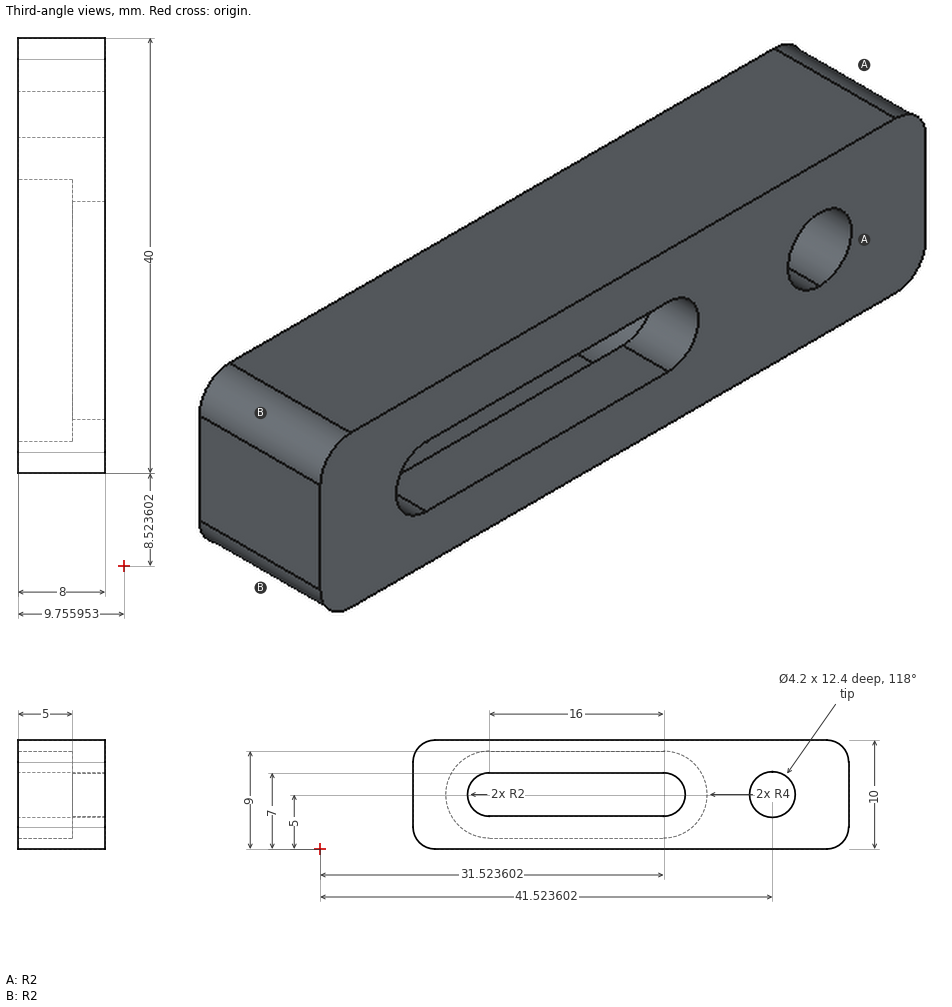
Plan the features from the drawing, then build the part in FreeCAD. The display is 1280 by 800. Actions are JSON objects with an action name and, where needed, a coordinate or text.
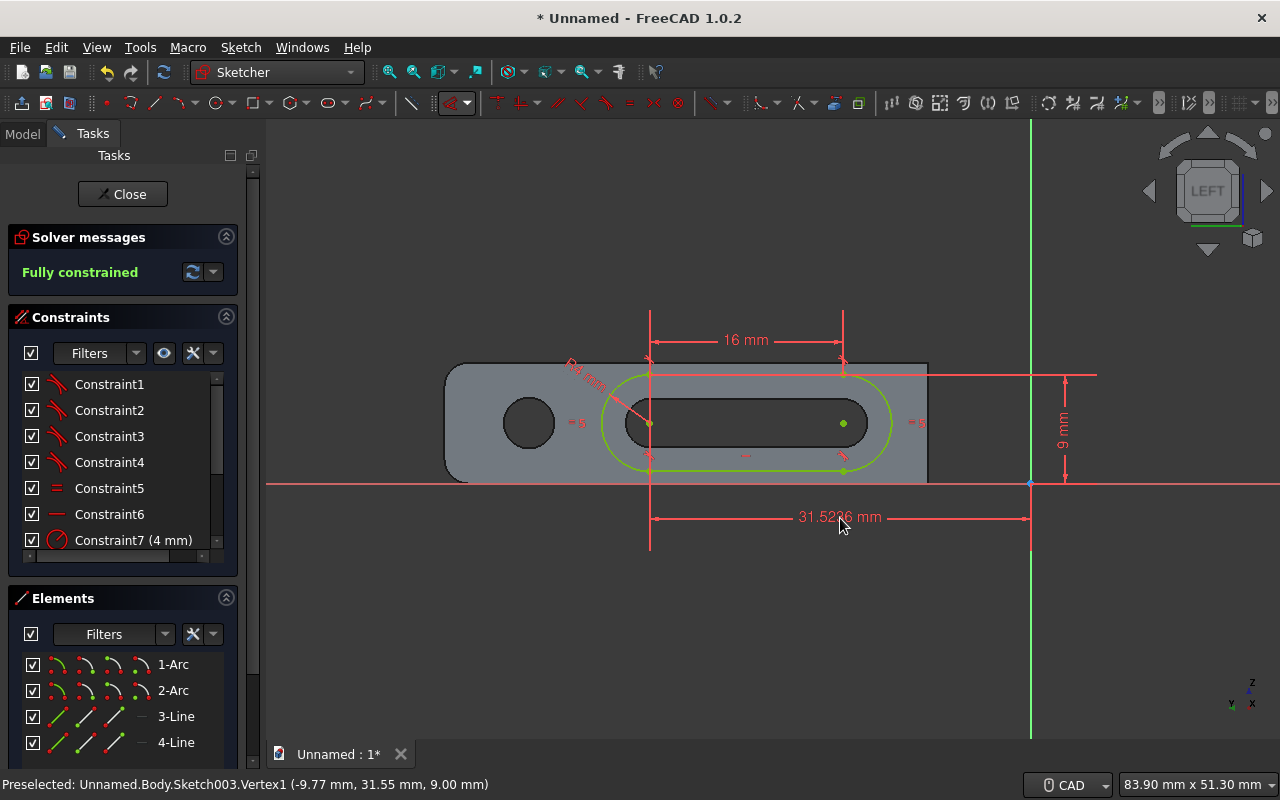
{"action": "left_click", "coordinate": [123, 194]}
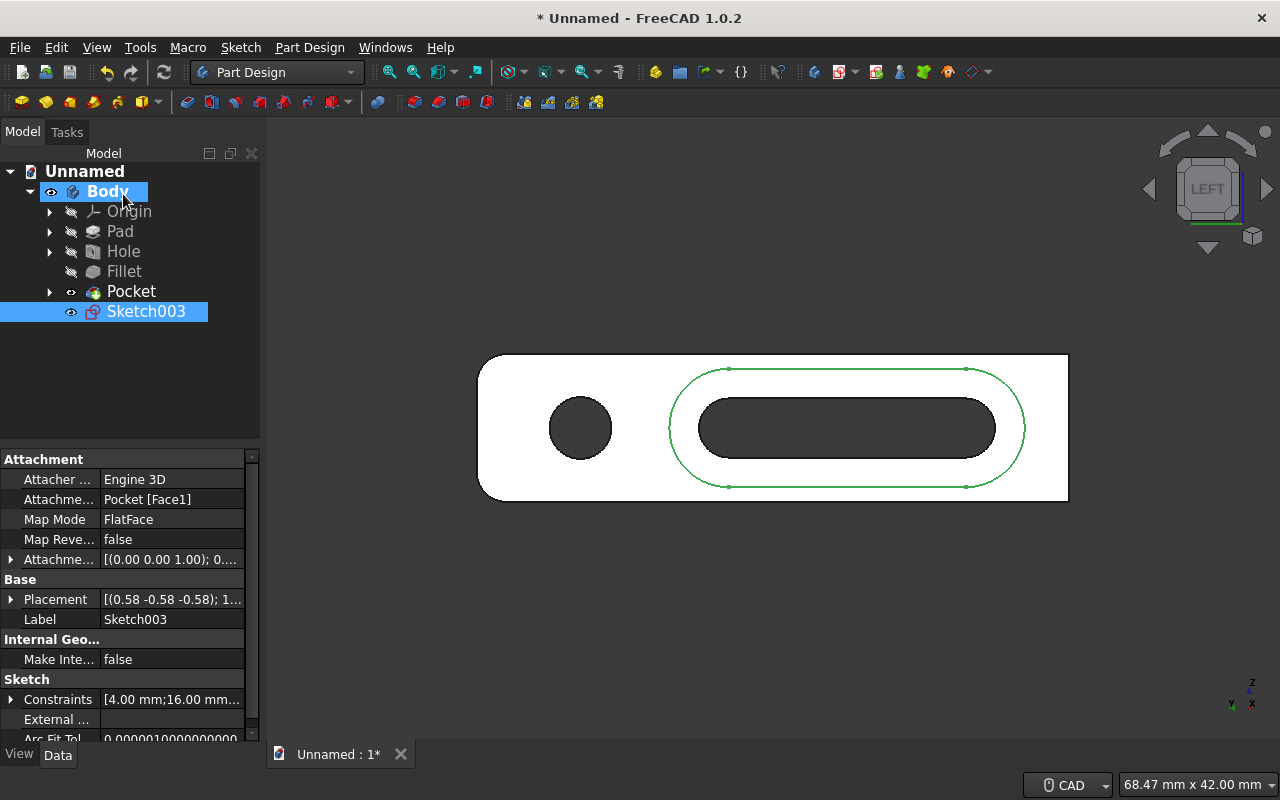
{"action": "left_click", "coordinate": [188, 102]}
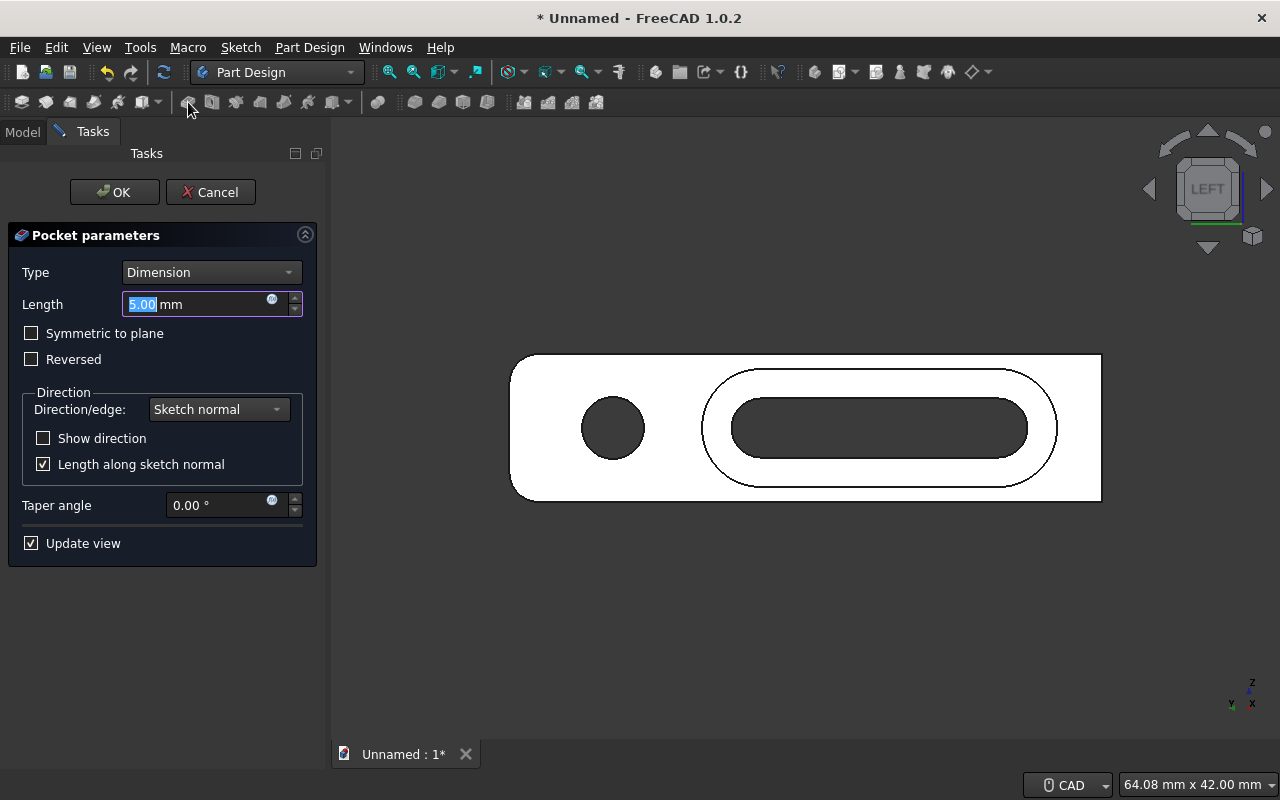
{"action": "type", "text": "5"}
{"action": "key", "text": "Tab"}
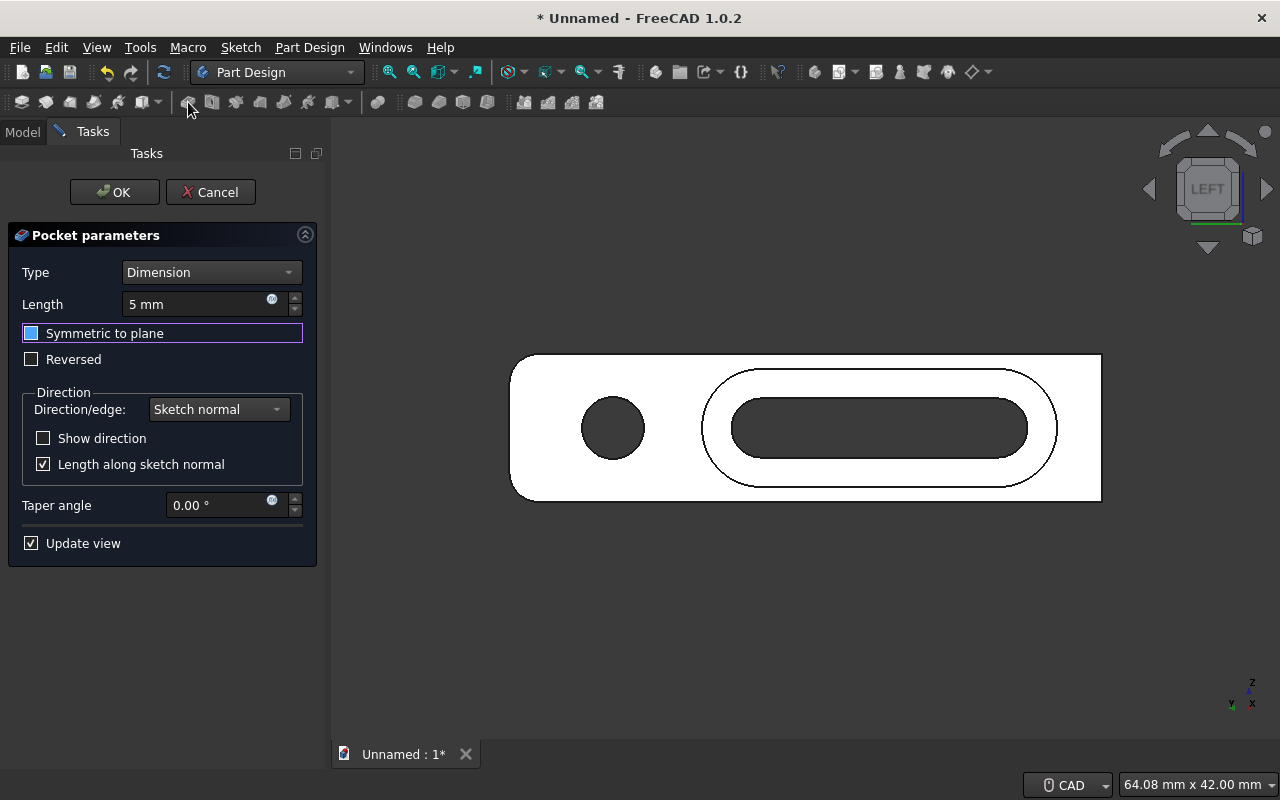
{"action": "left_click", "coordinate": [115, 192]}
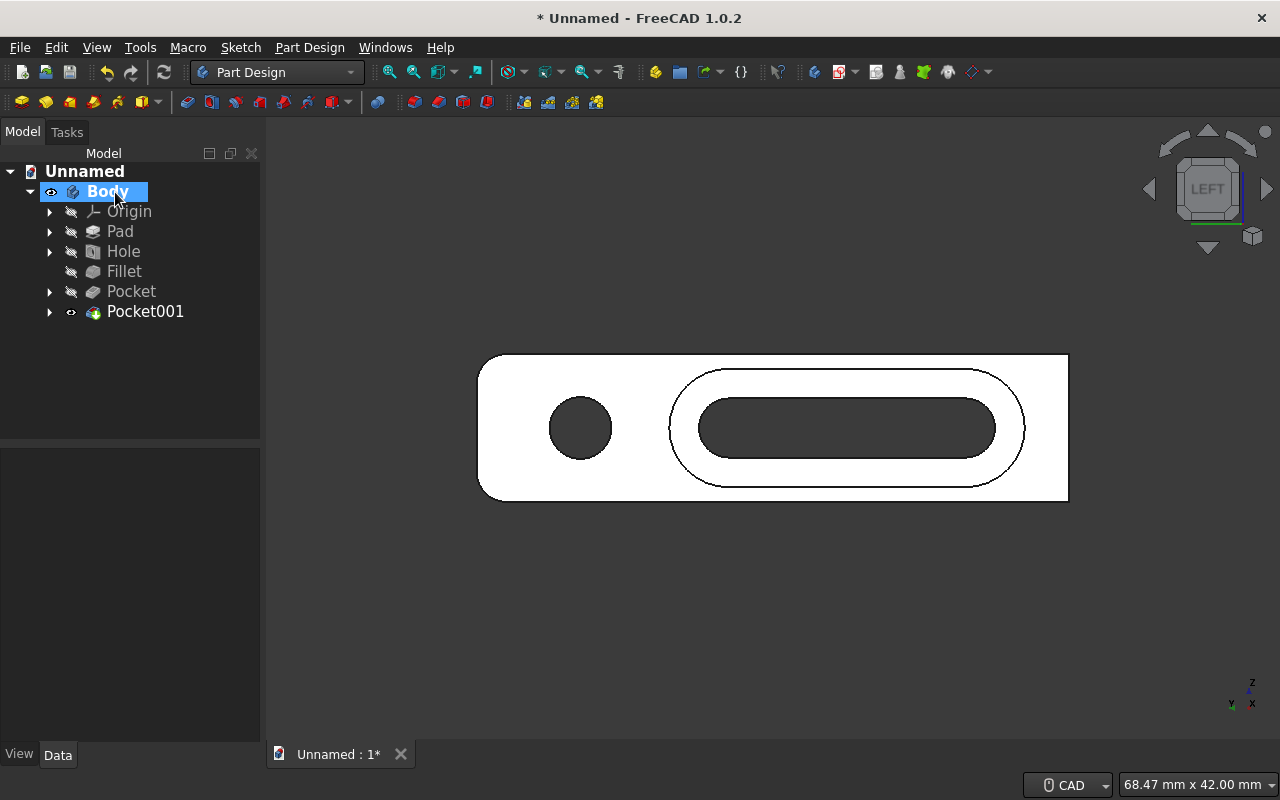
{"action": "key", "text": "0"}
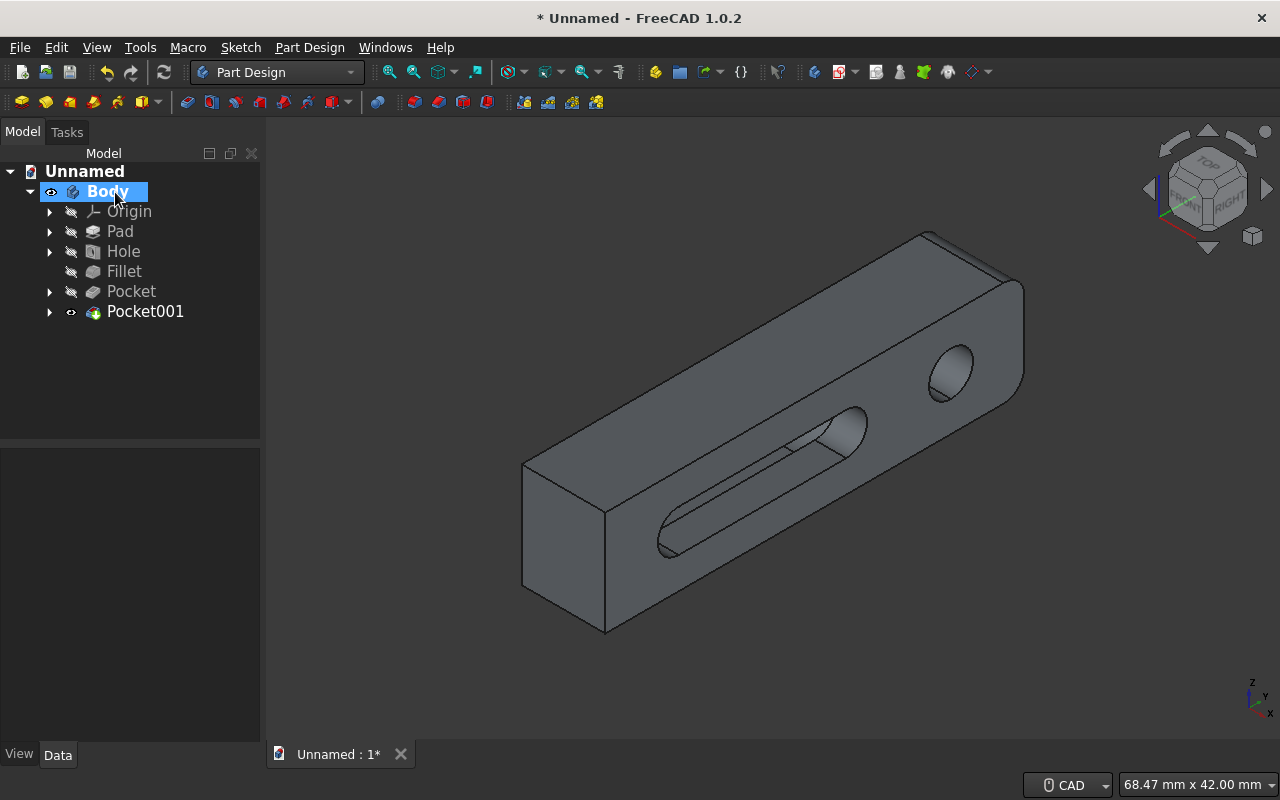
{"action": "left_click", "coordinate": [564, 487]}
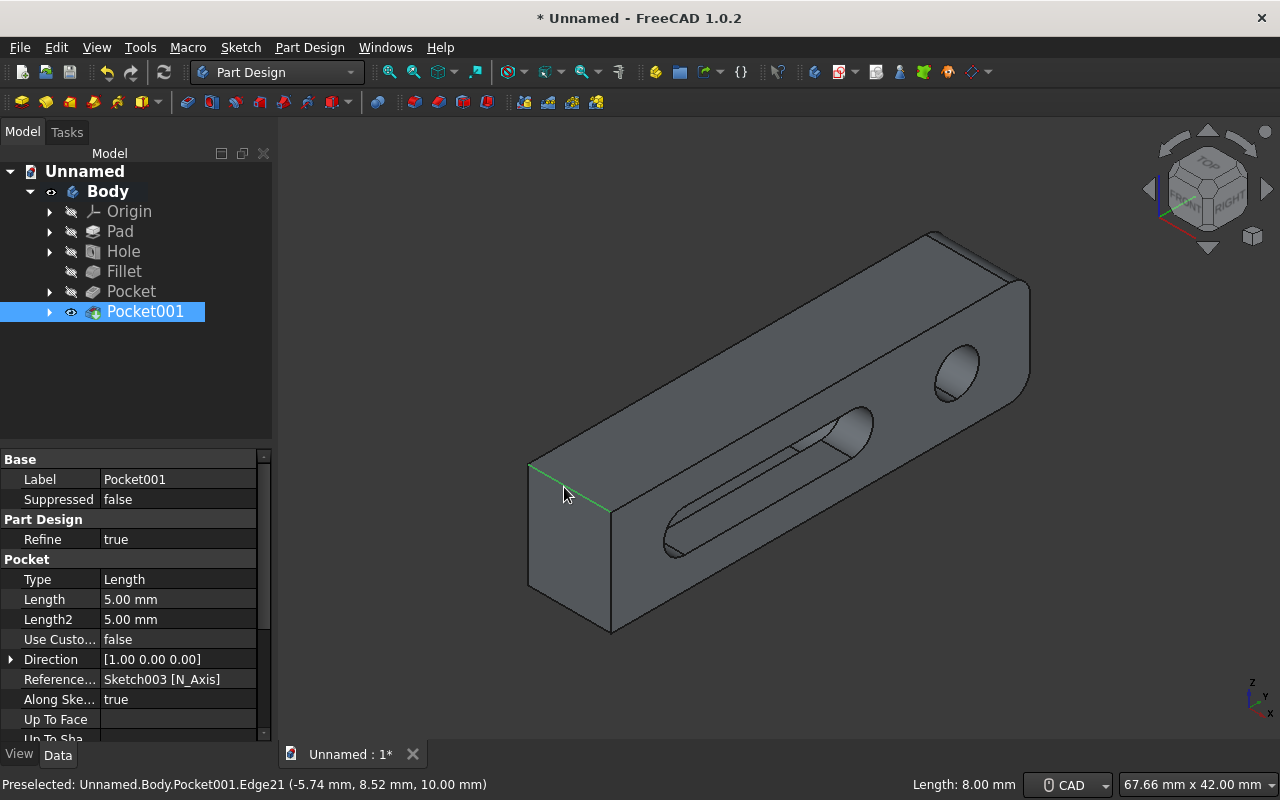
{"action": "key", "text": "2"}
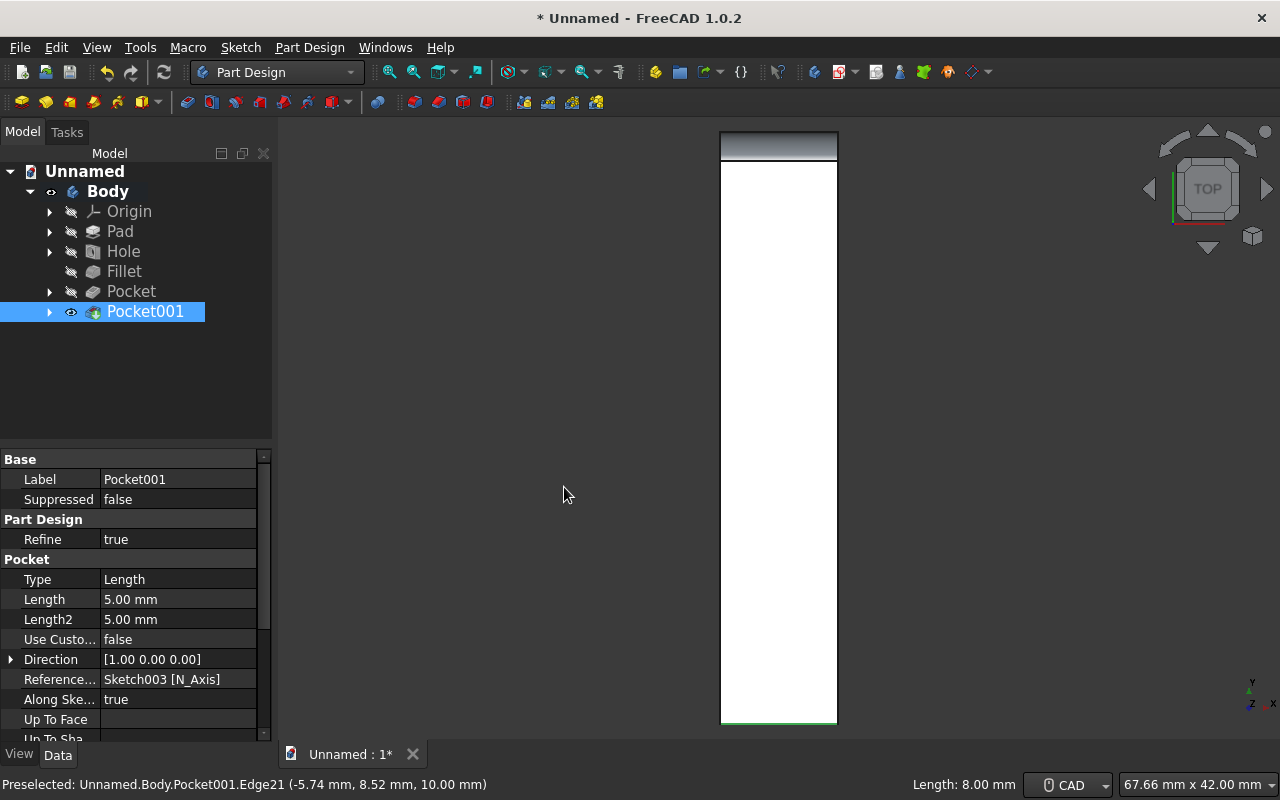
{"action": "key", "text": "1"}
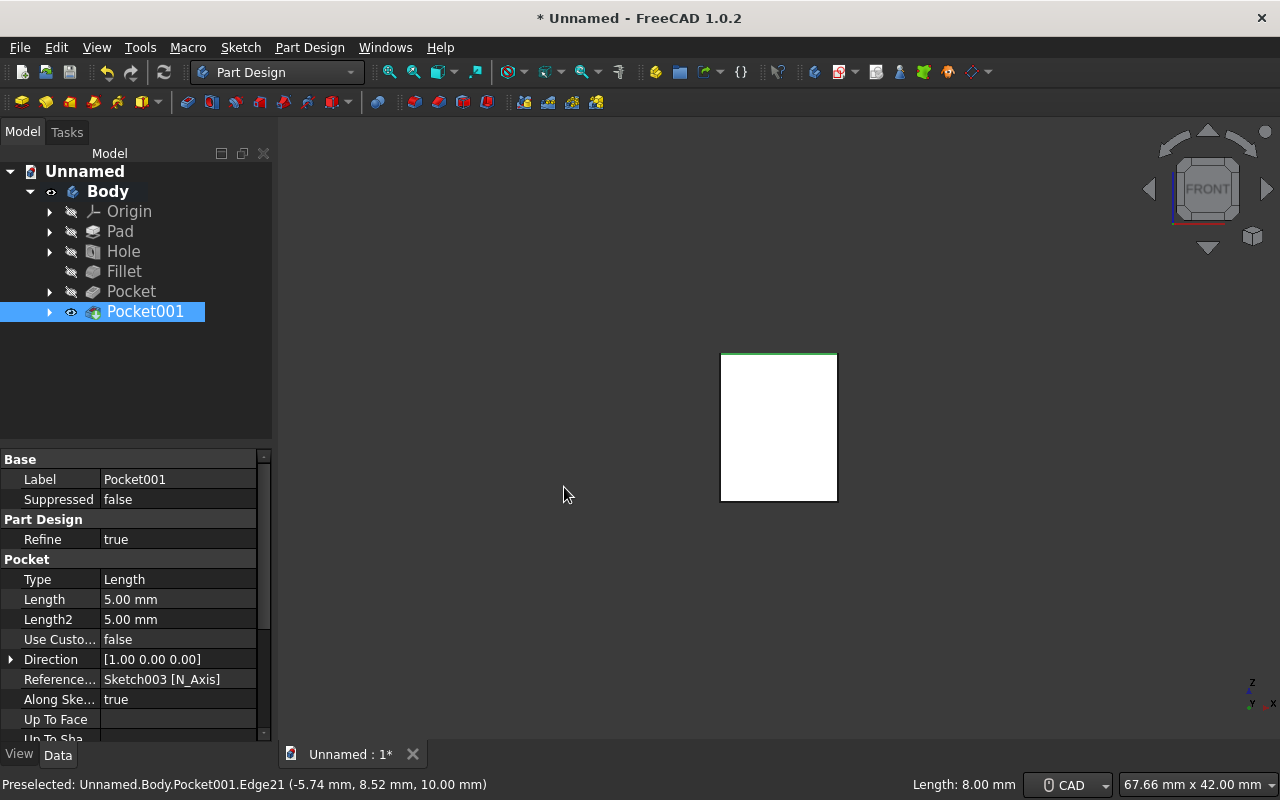
{"action": "key", "text": "v f"}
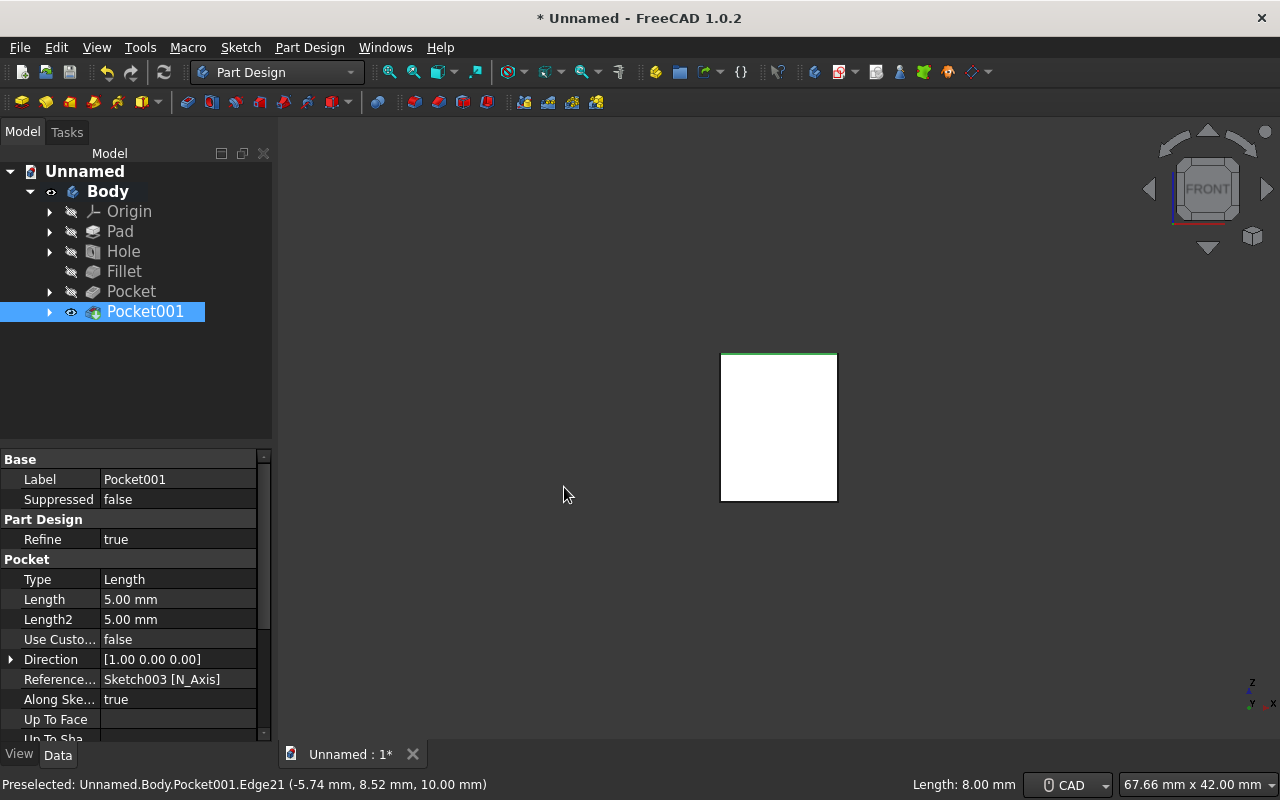
{"action": "left_click", "coordinate": [779, 501], "text": "ctrl"}